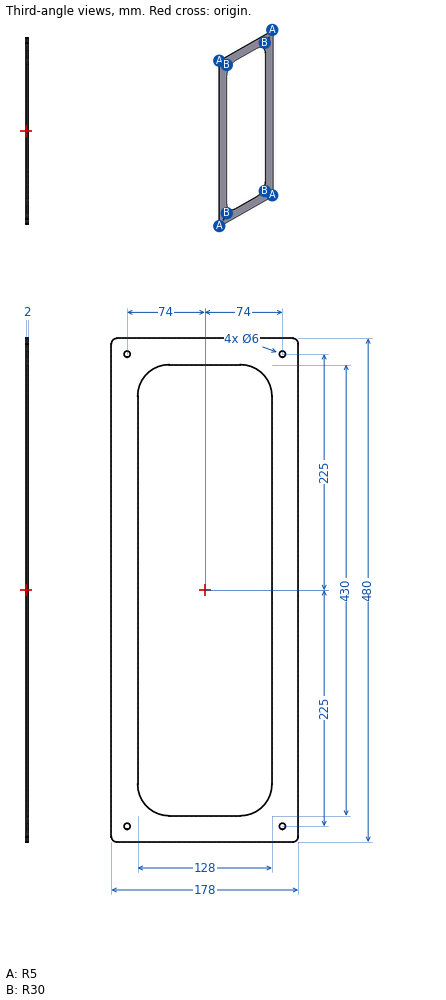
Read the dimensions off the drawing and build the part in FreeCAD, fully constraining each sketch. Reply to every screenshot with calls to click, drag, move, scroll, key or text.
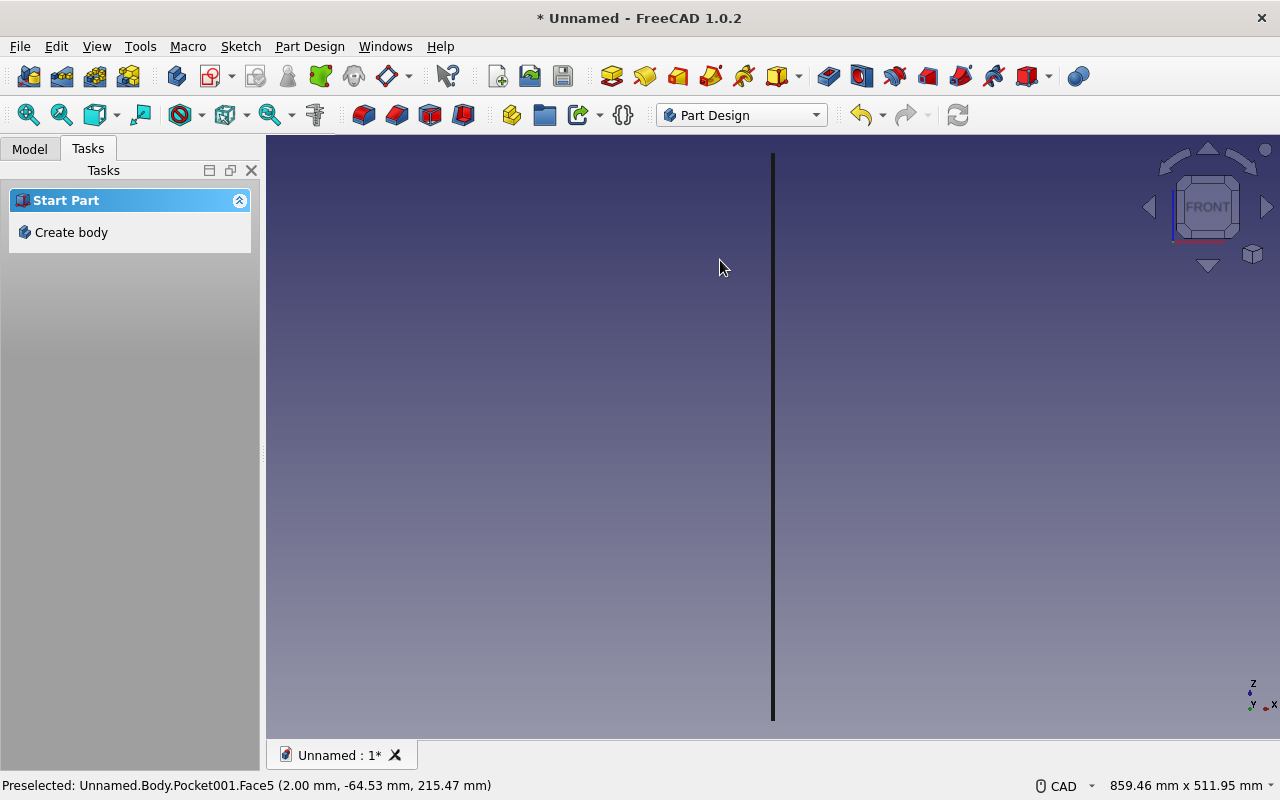
scroll(773, 182, up, 15)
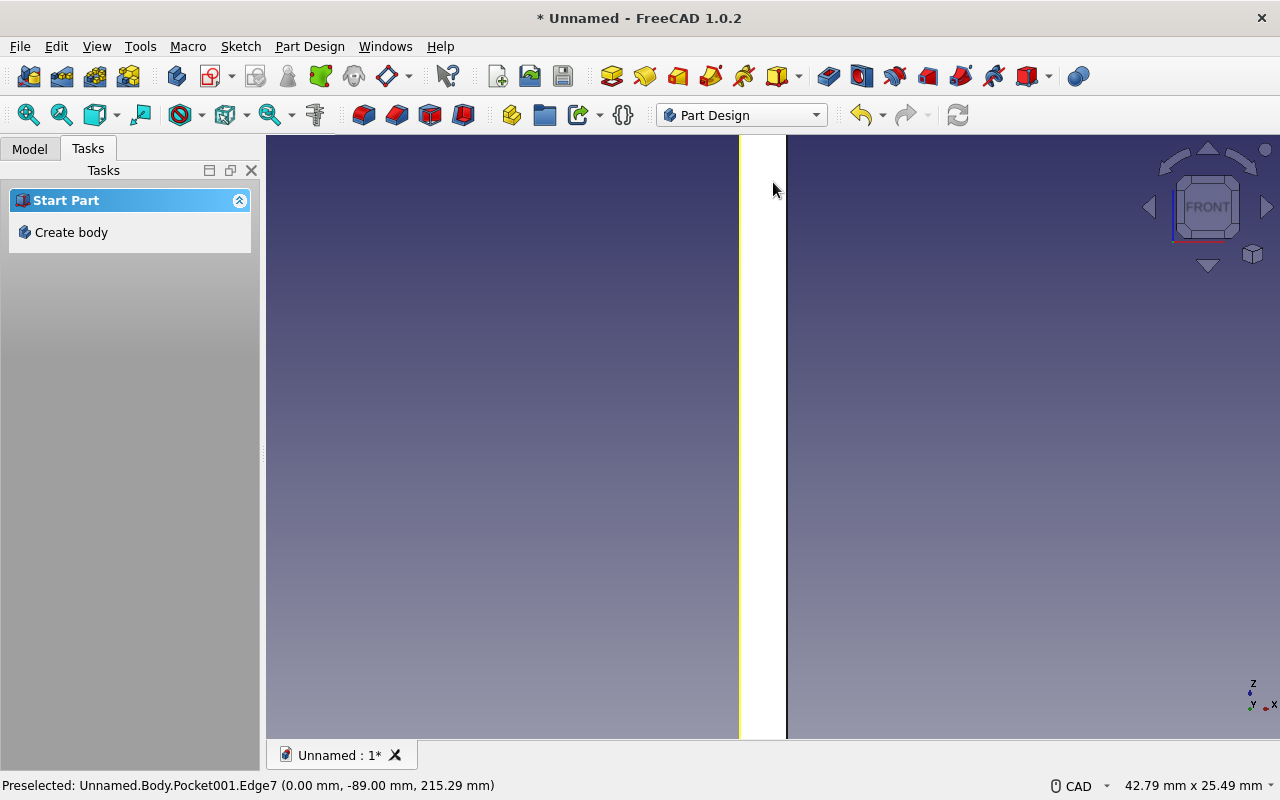
click(29, 116)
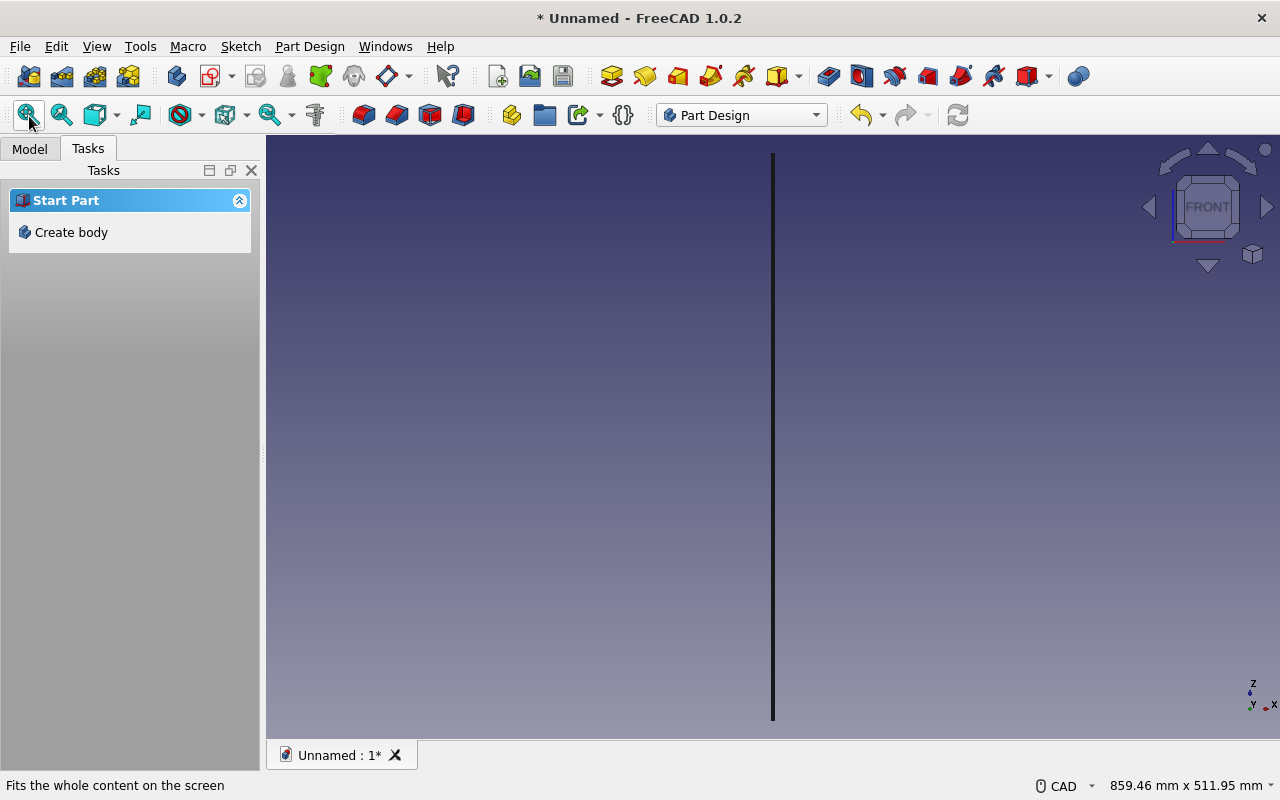
key(3)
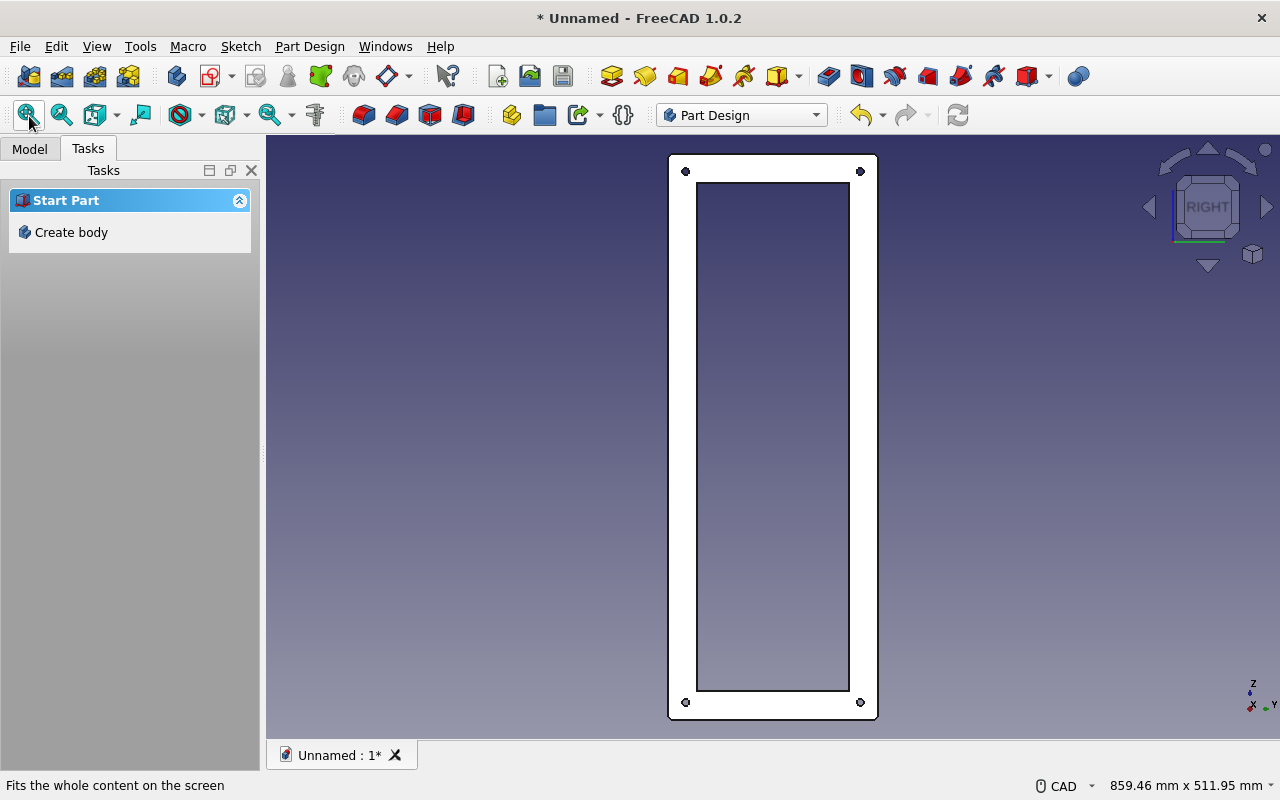
scroll(697, 182, up, 15)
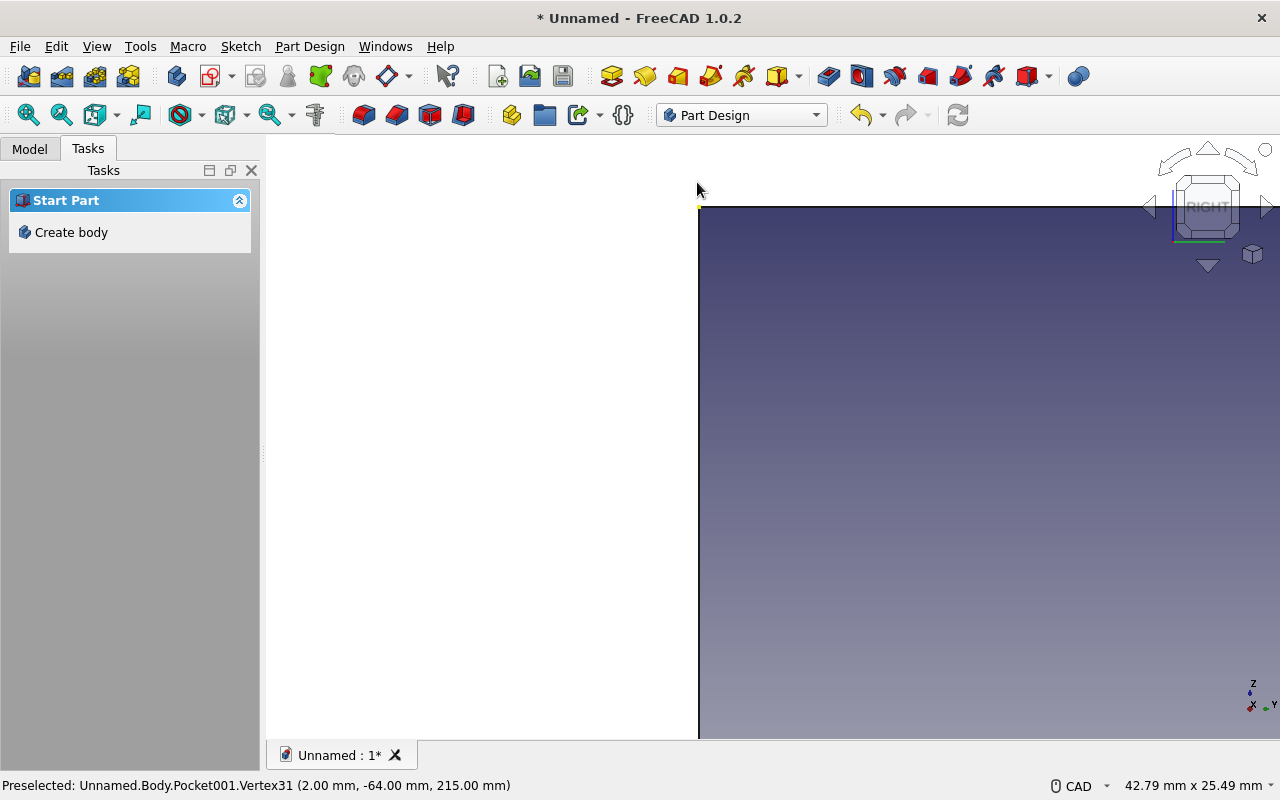
key(v)
key(f)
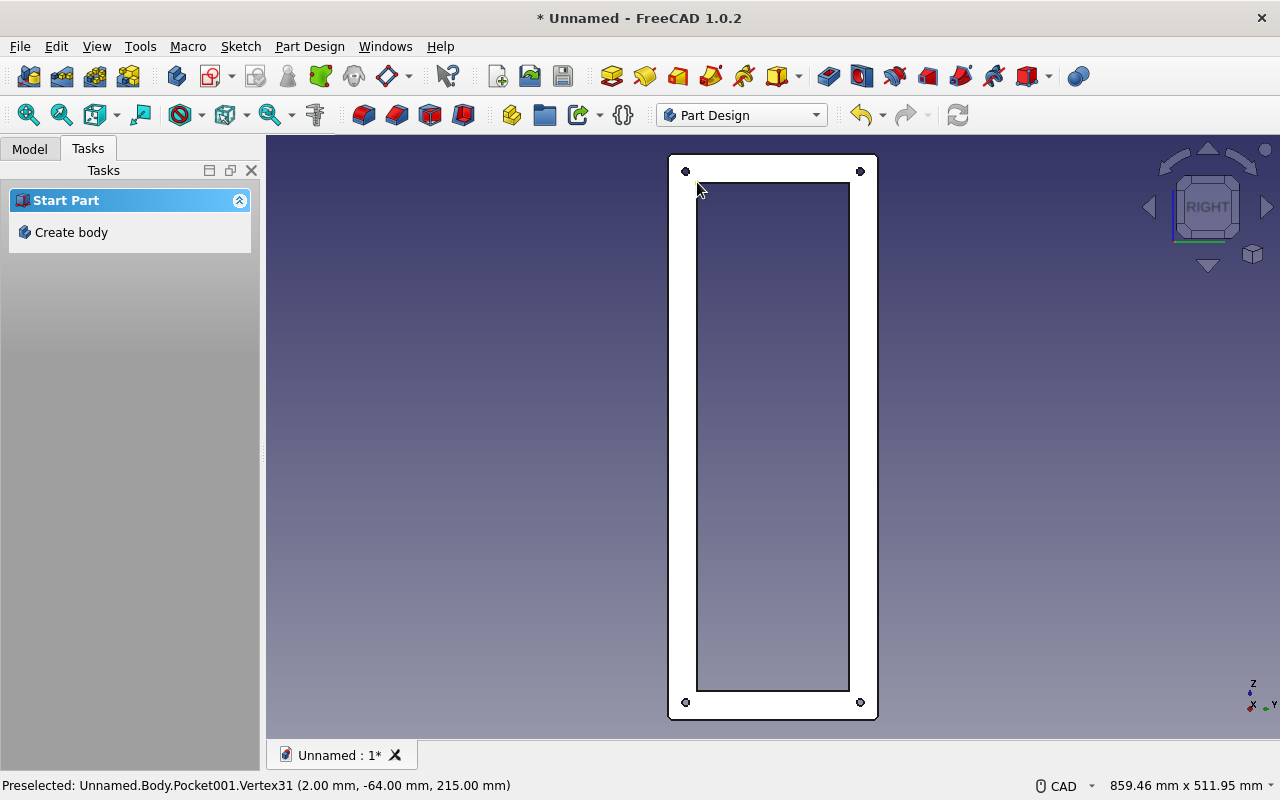
key(5)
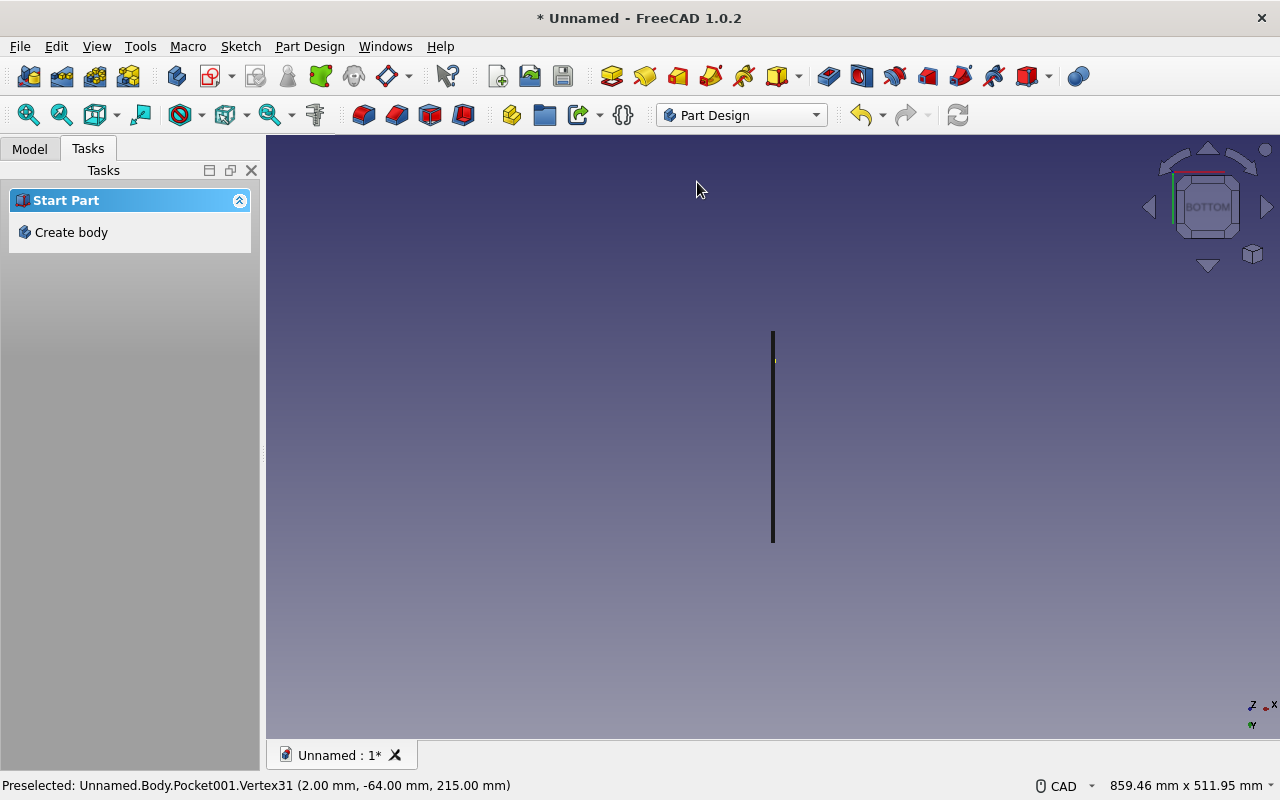
key(v)
key(f)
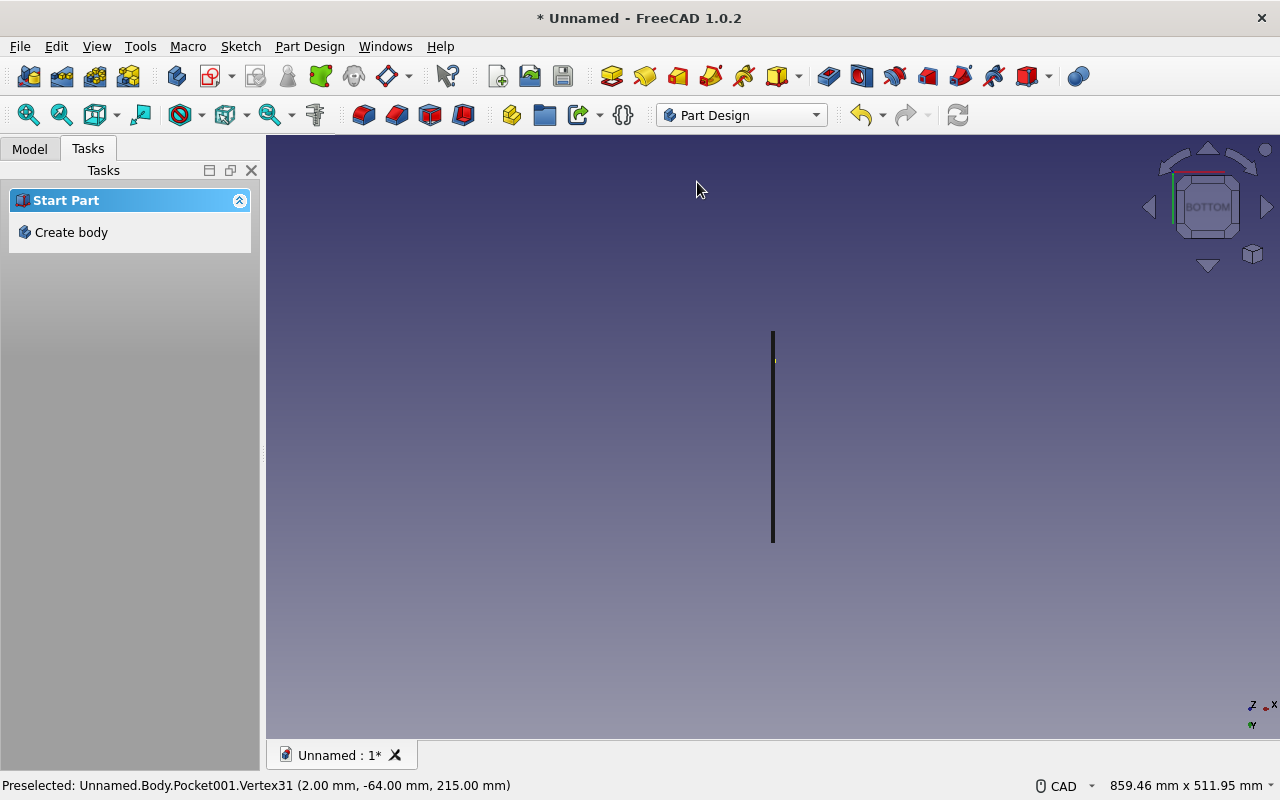
scroll(773, 360, up, 15)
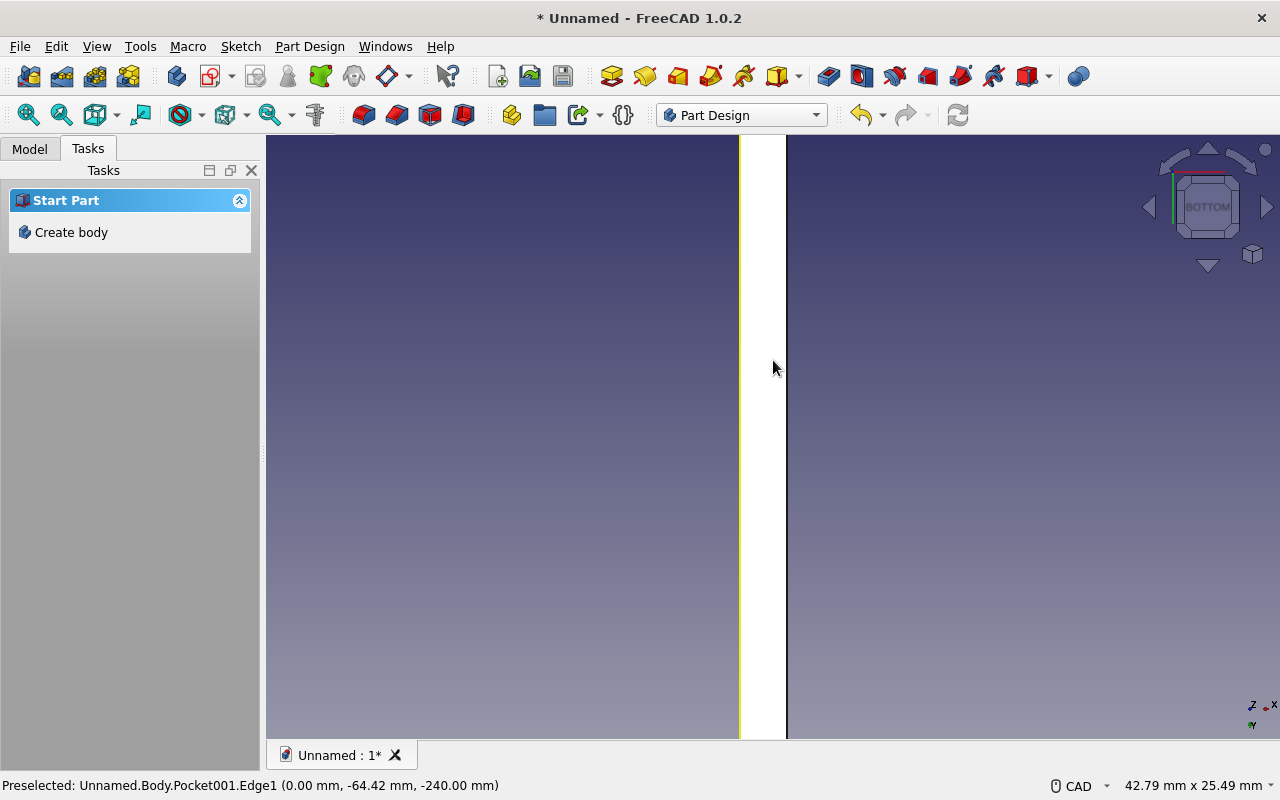
key(v)
key(f)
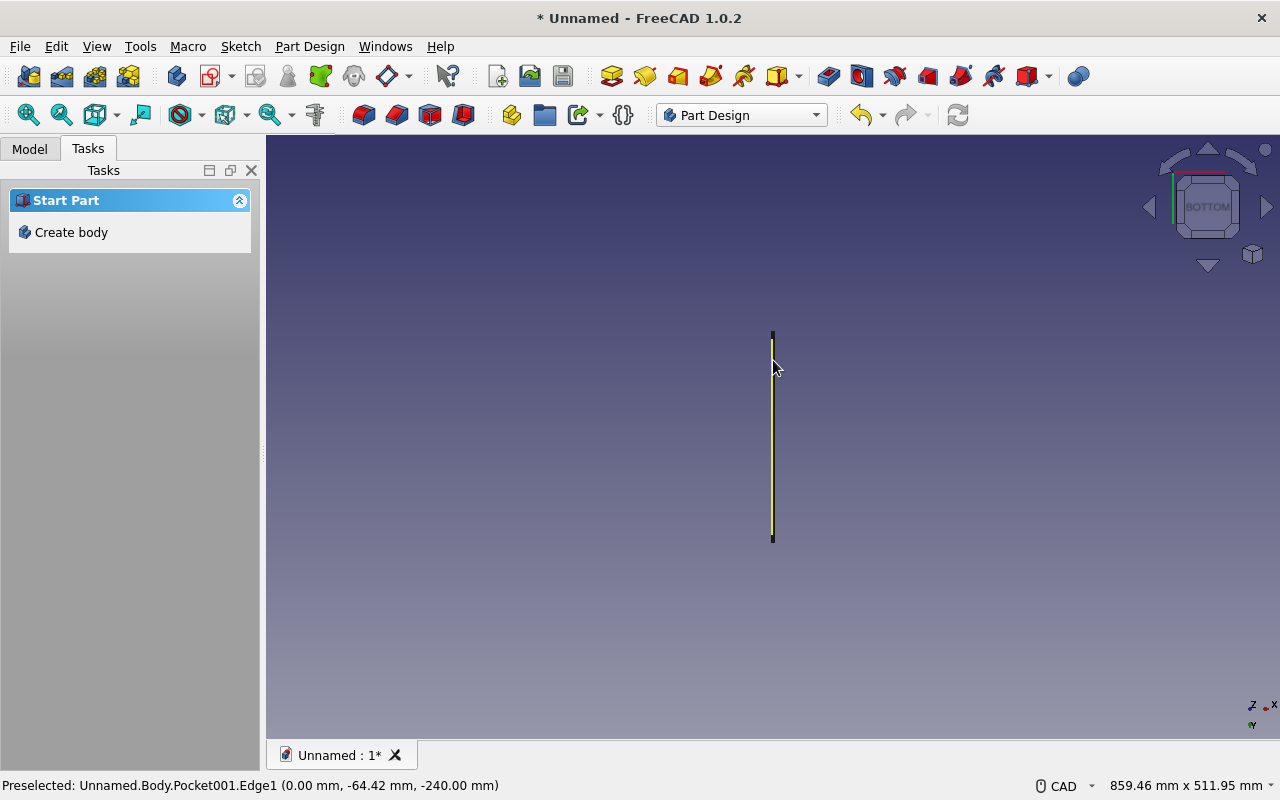
key(4)